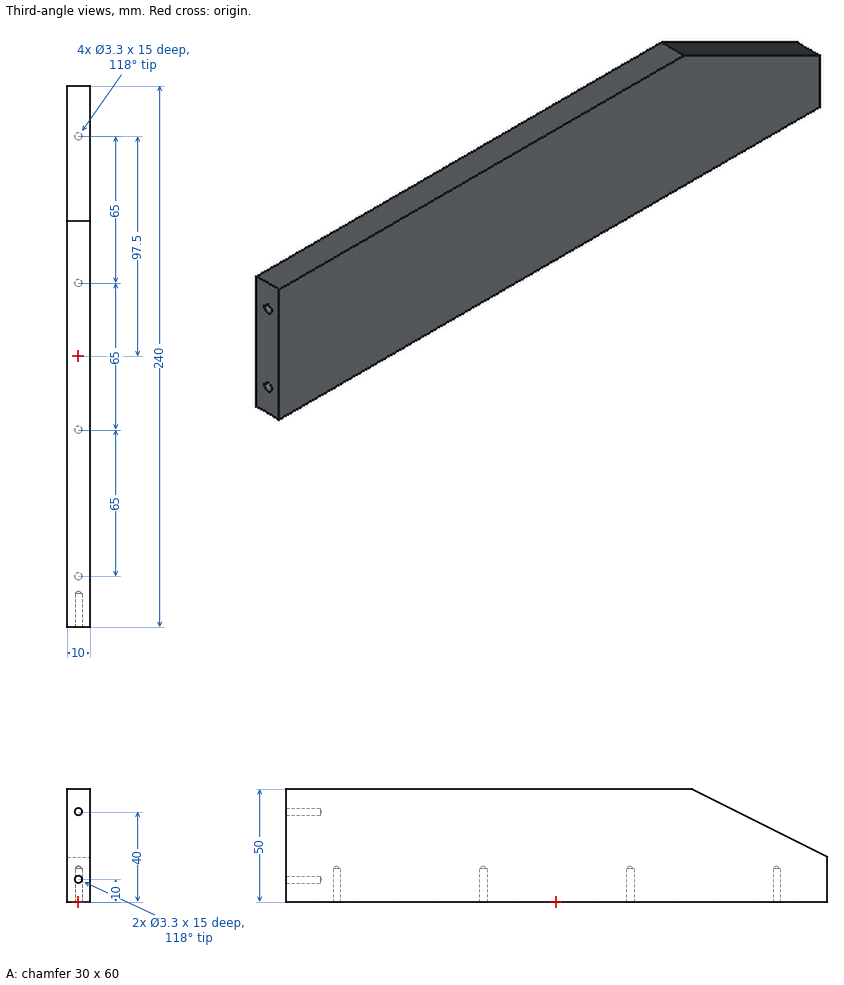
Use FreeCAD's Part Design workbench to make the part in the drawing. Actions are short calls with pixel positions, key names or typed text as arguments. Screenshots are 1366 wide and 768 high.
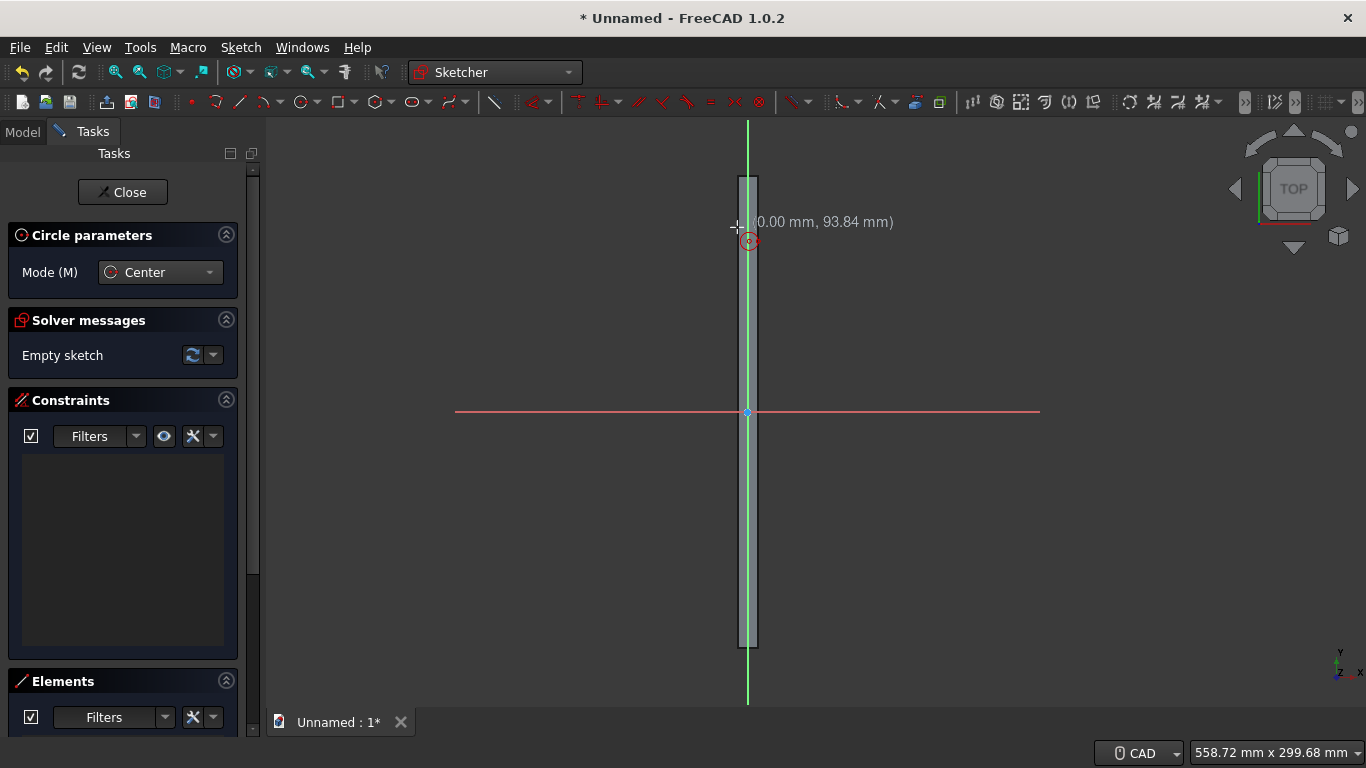
click(748, 220)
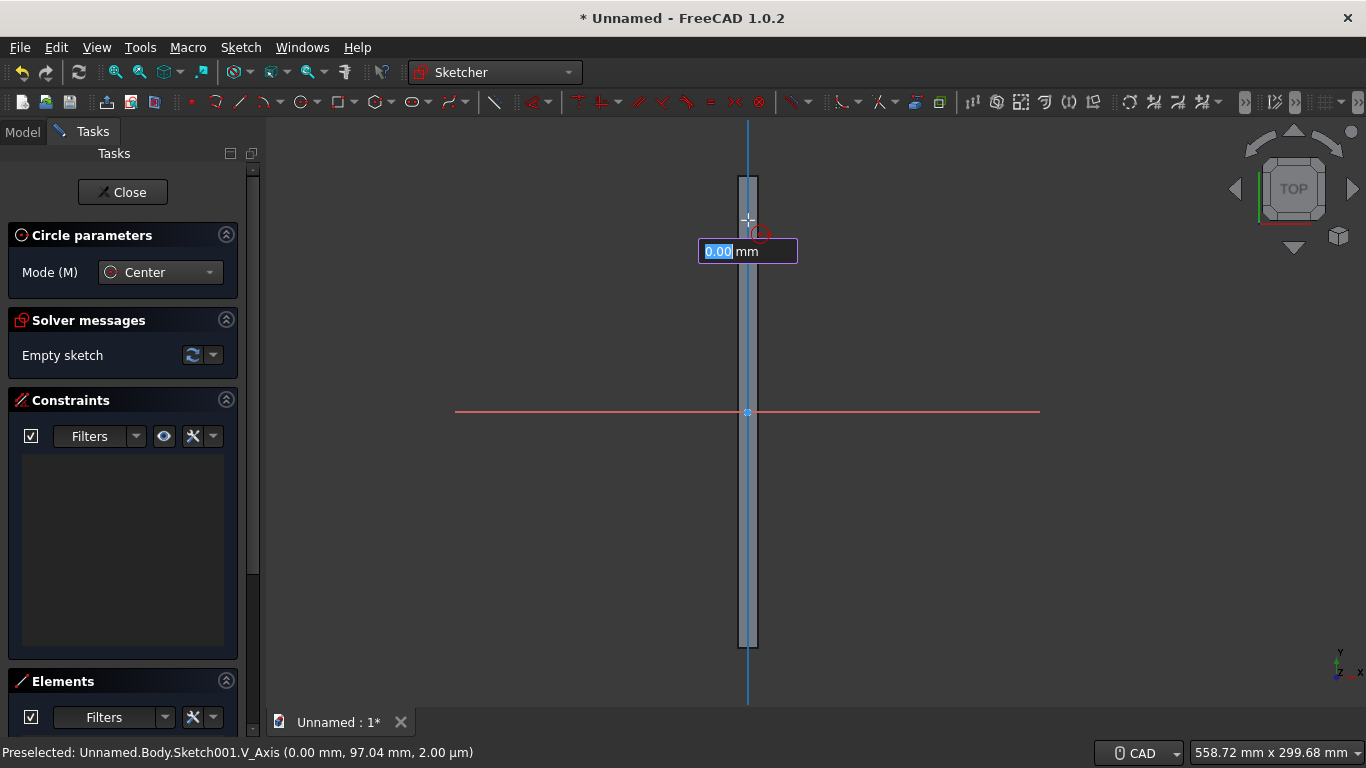
scroll(751, 219, up, 9)
move(747, 218)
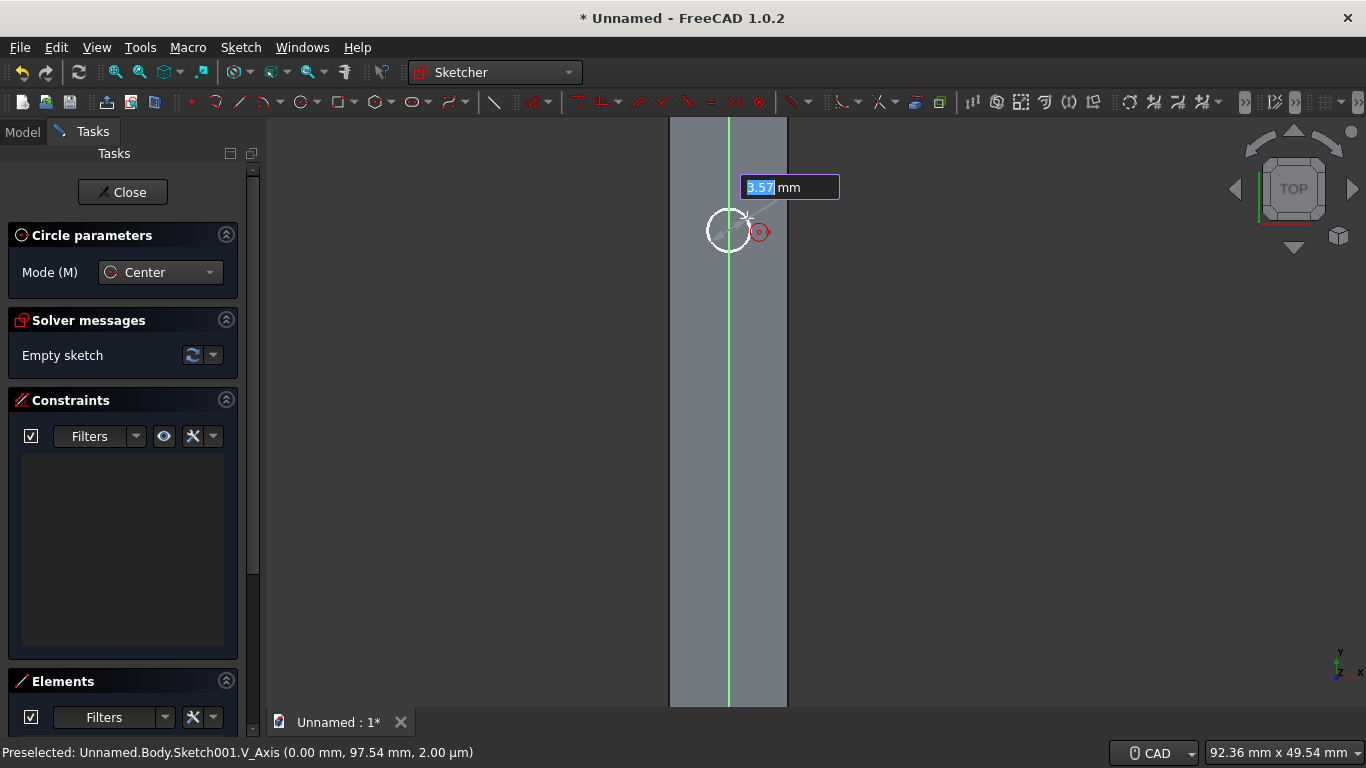
text(3.3)
key(Return)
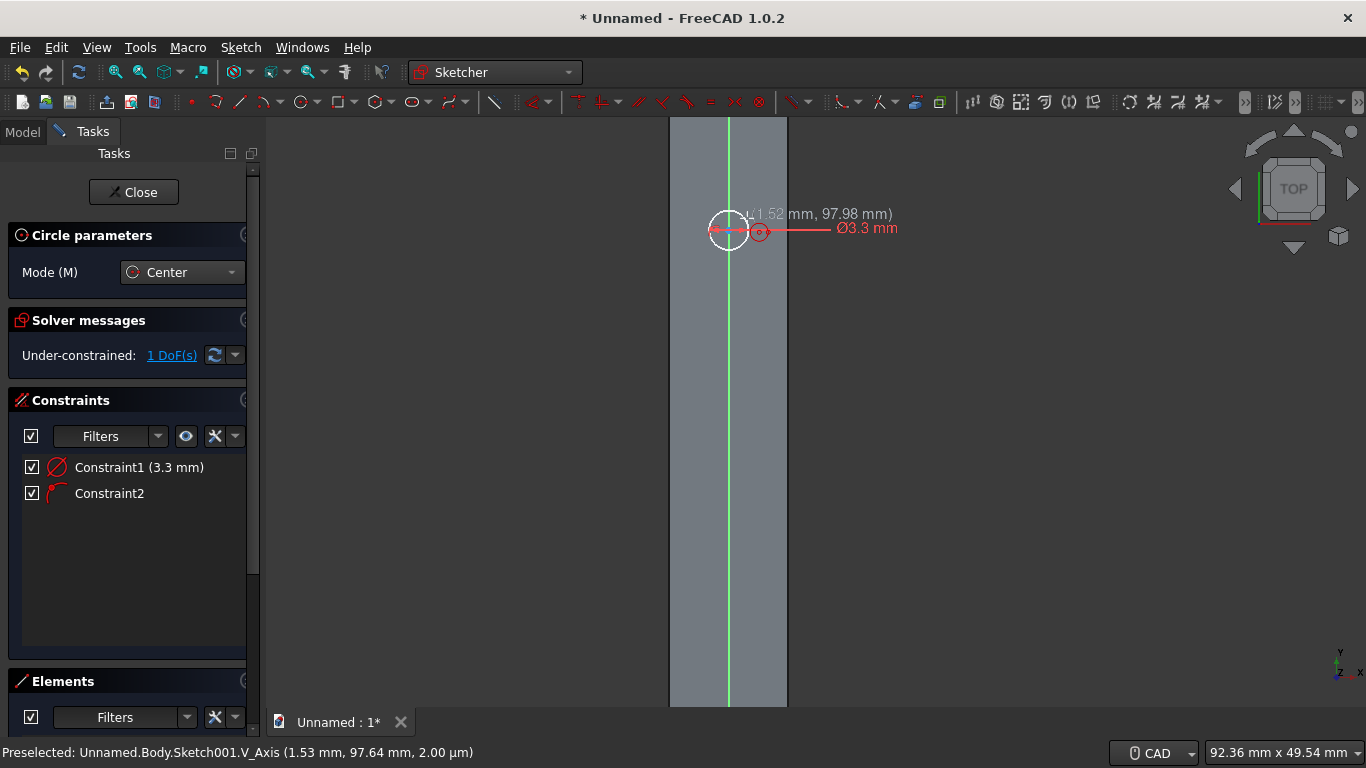
scroll(751, 219, down, 9)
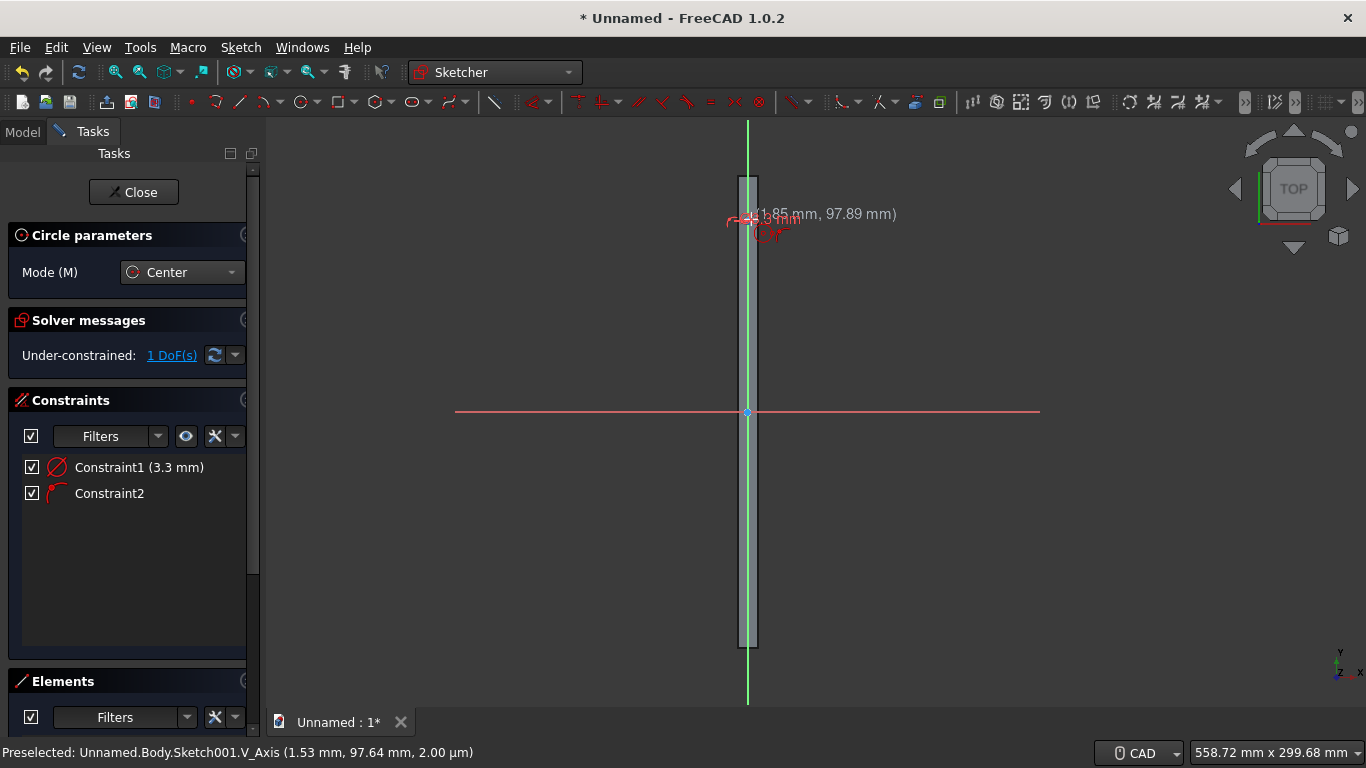
scroll(748, 348, up, 10)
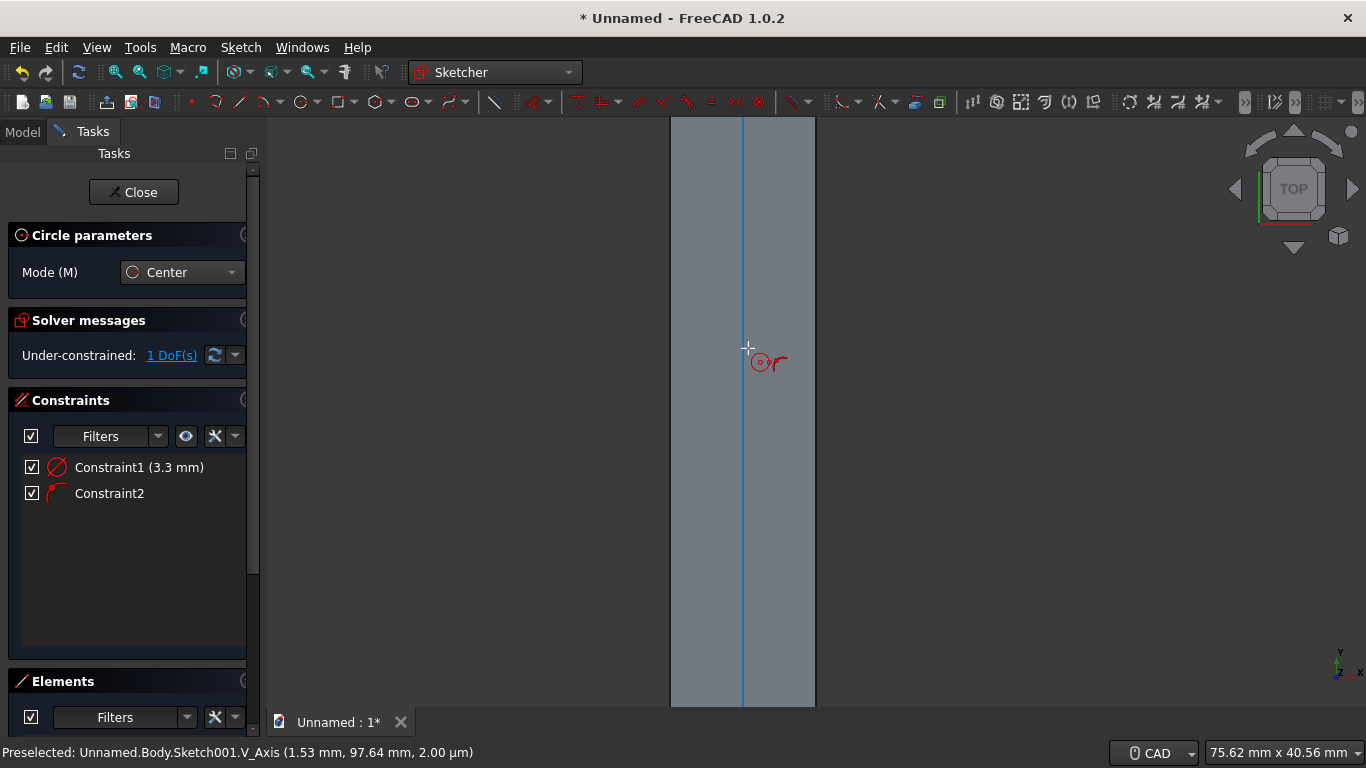
scroll(748, 348, down, 10)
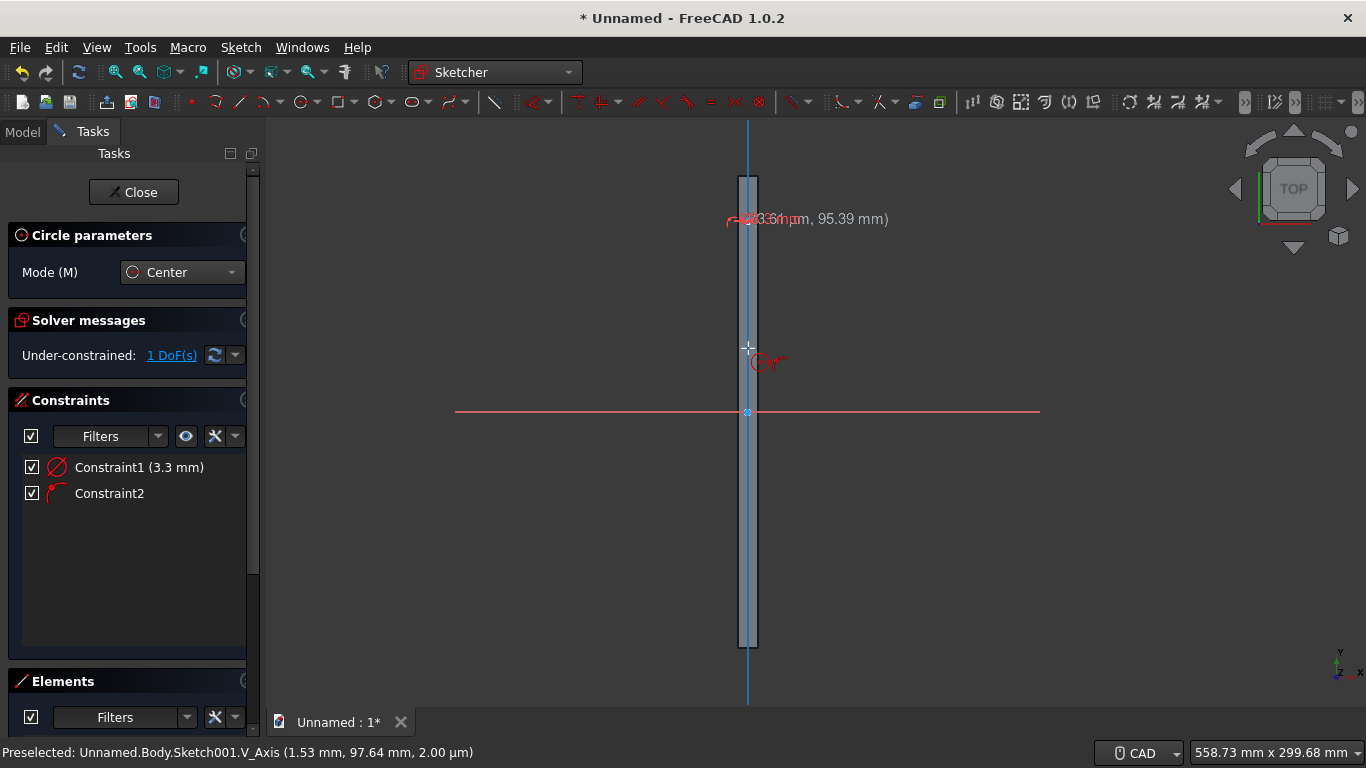
click(748, 348)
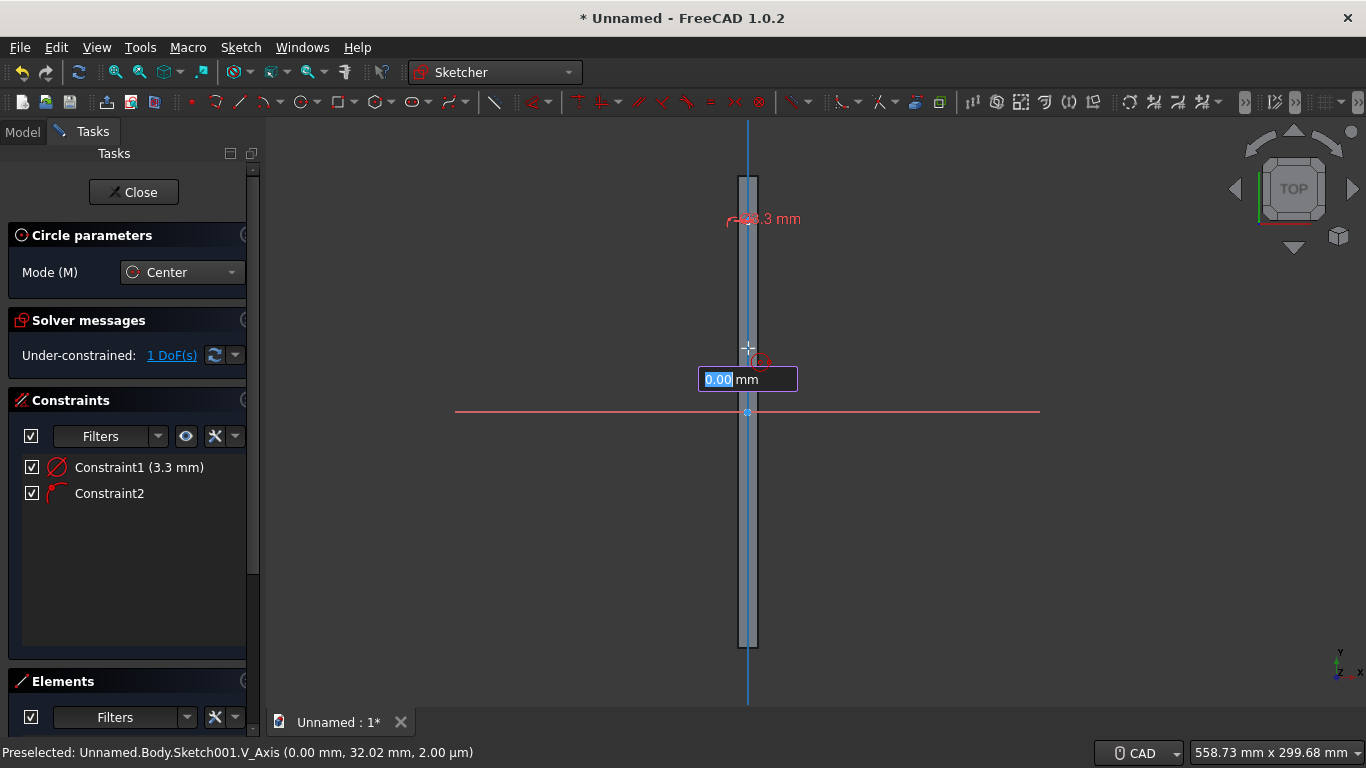
scroll(751, 347, up, 9)
move(747, 345)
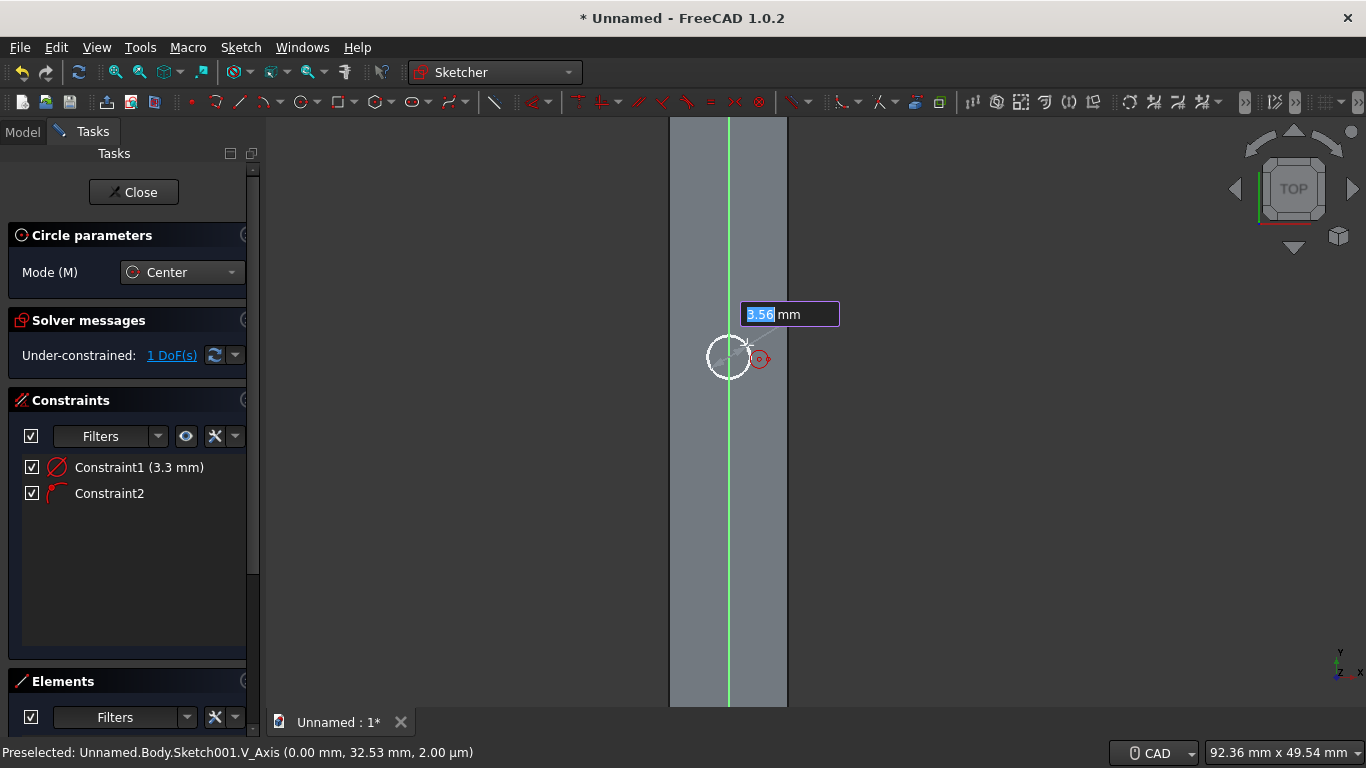
text(3.3)
key(Return)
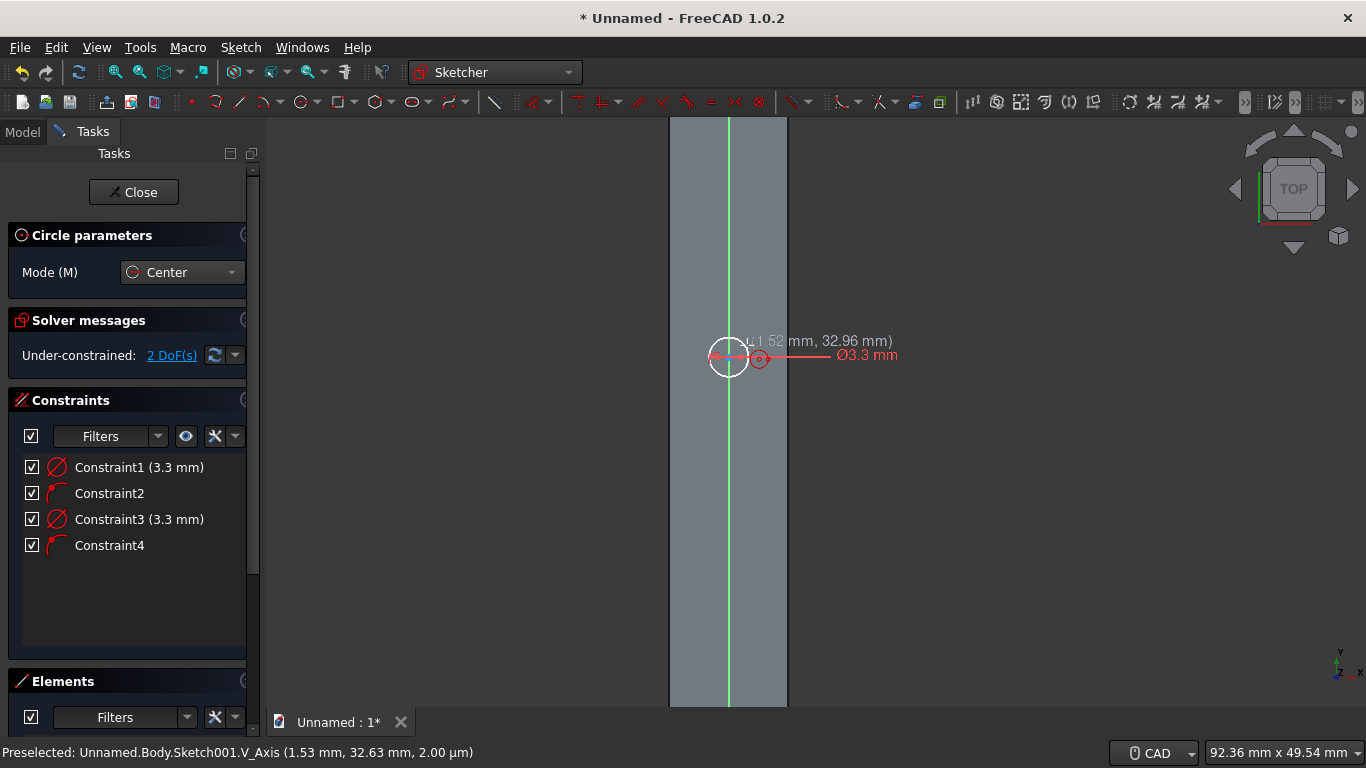
scroll(751, 347, down, 9)